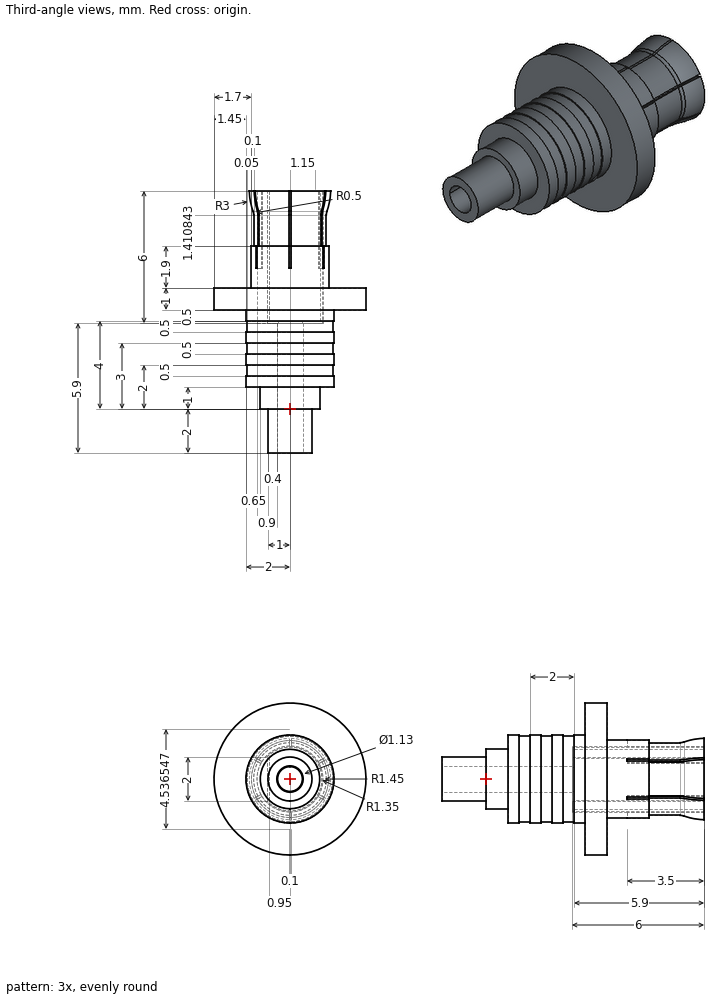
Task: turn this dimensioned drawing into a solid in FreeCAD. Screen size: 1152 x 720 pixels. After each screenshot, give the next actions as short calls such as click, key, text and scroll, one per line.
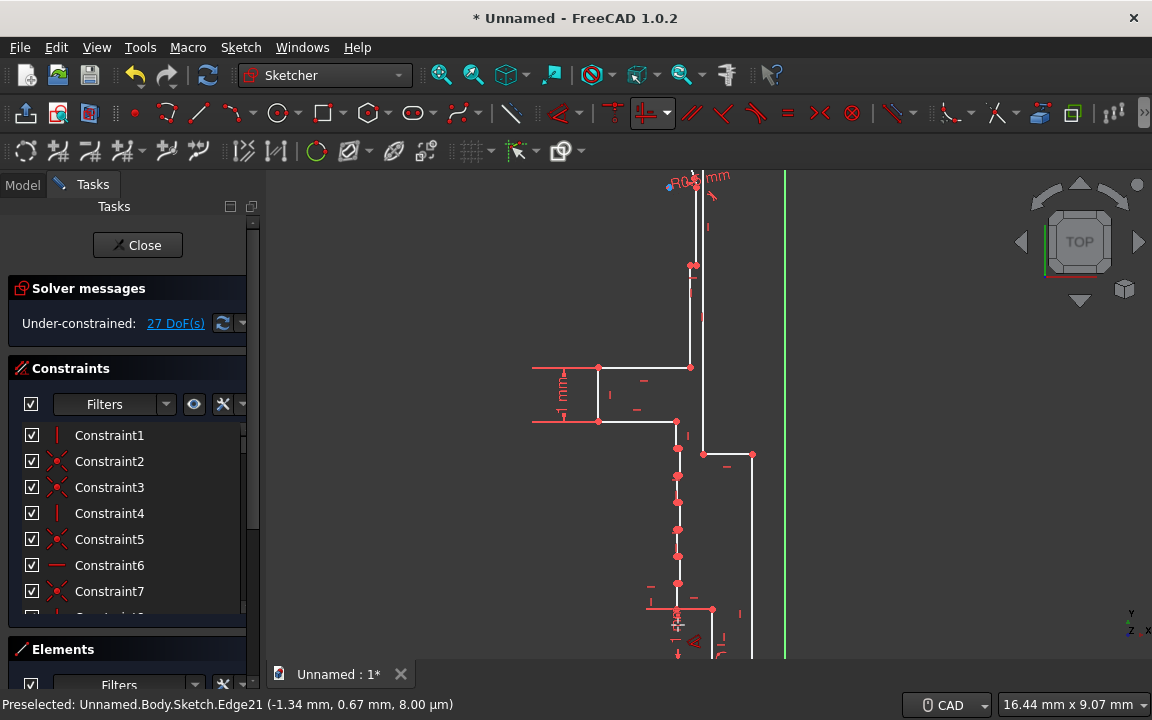
scroll(599, 385, down, 4)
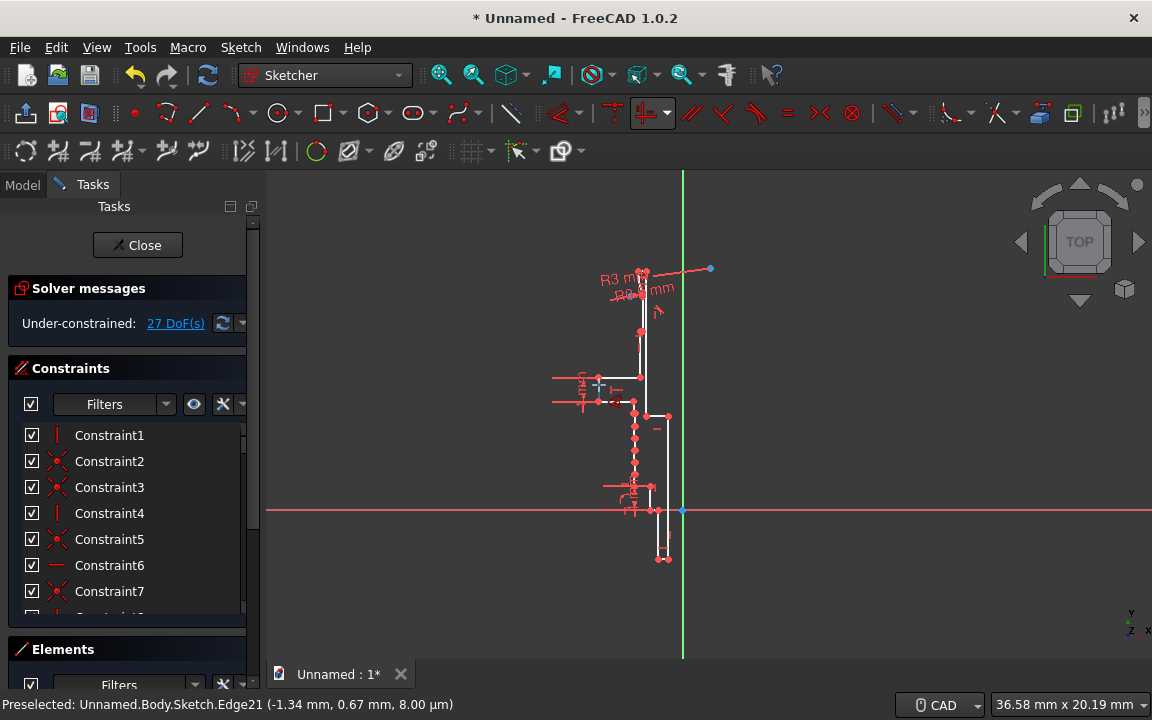
scroll(658, 525, up, 2)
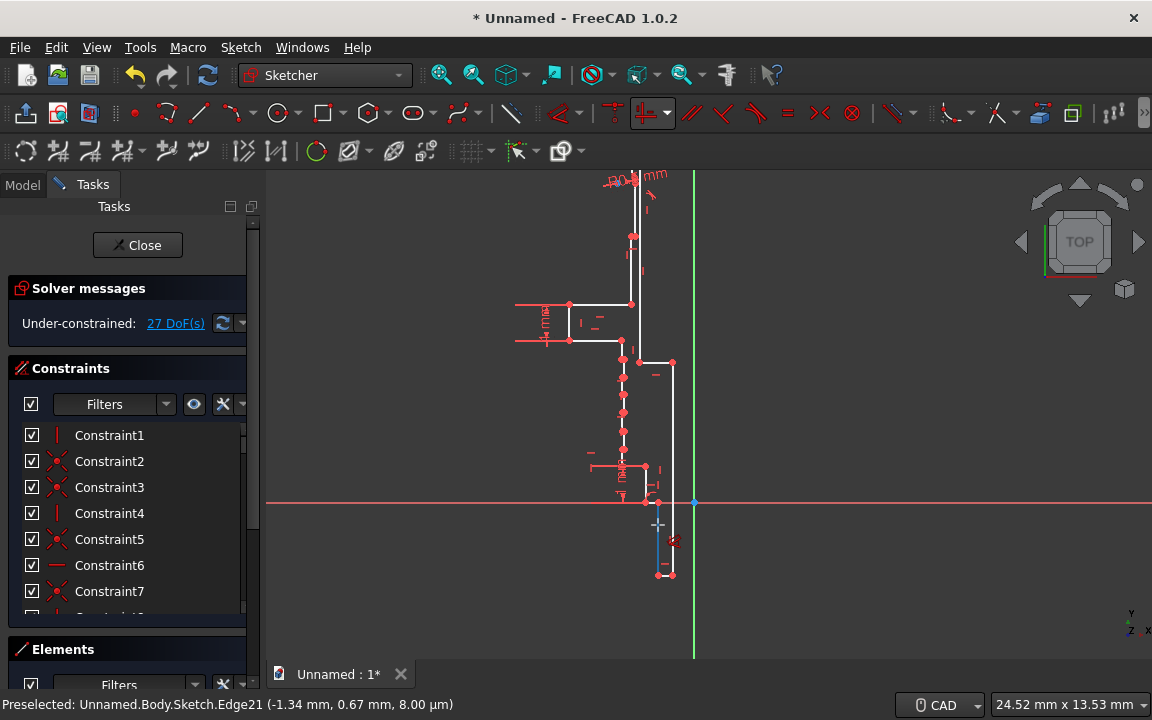
click(658, 525)
click(624, 539)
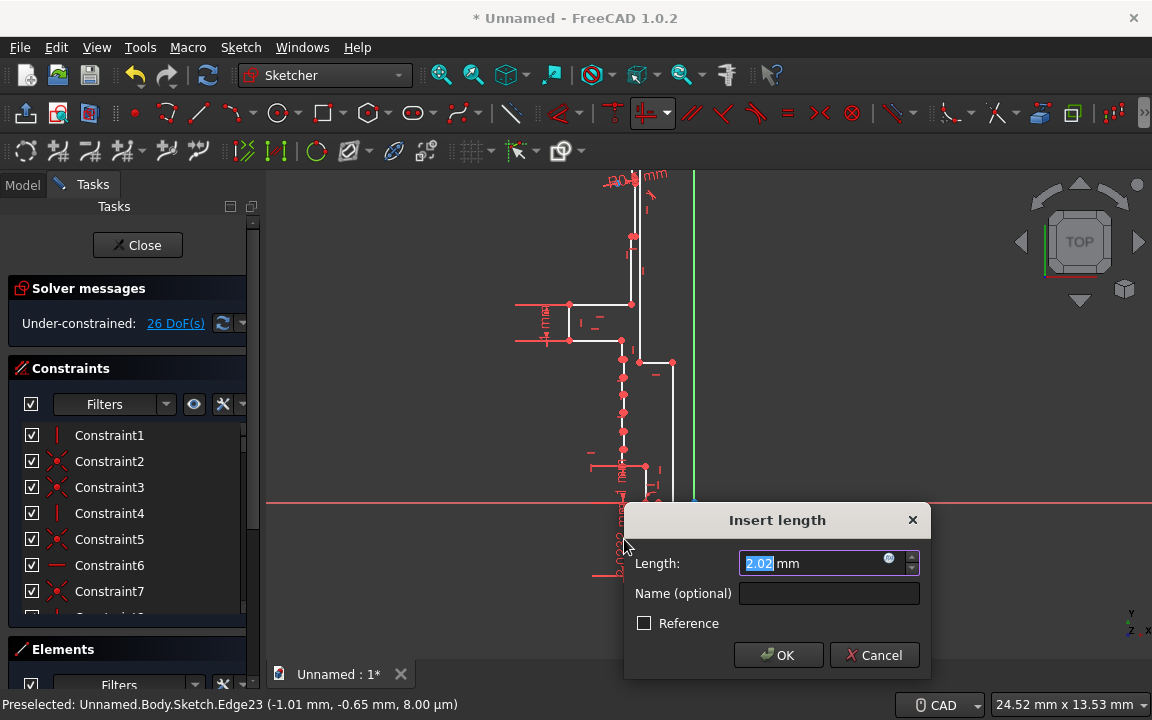
text(2)
key(Return)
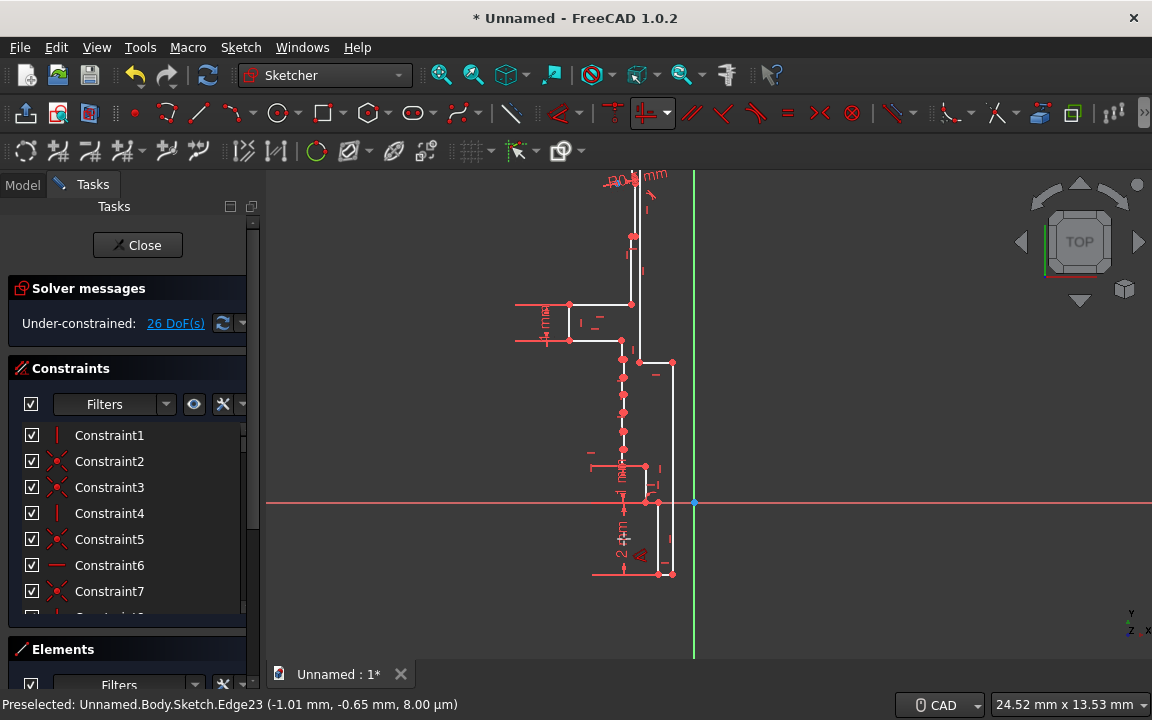
click(640, 319)
click(674, 280)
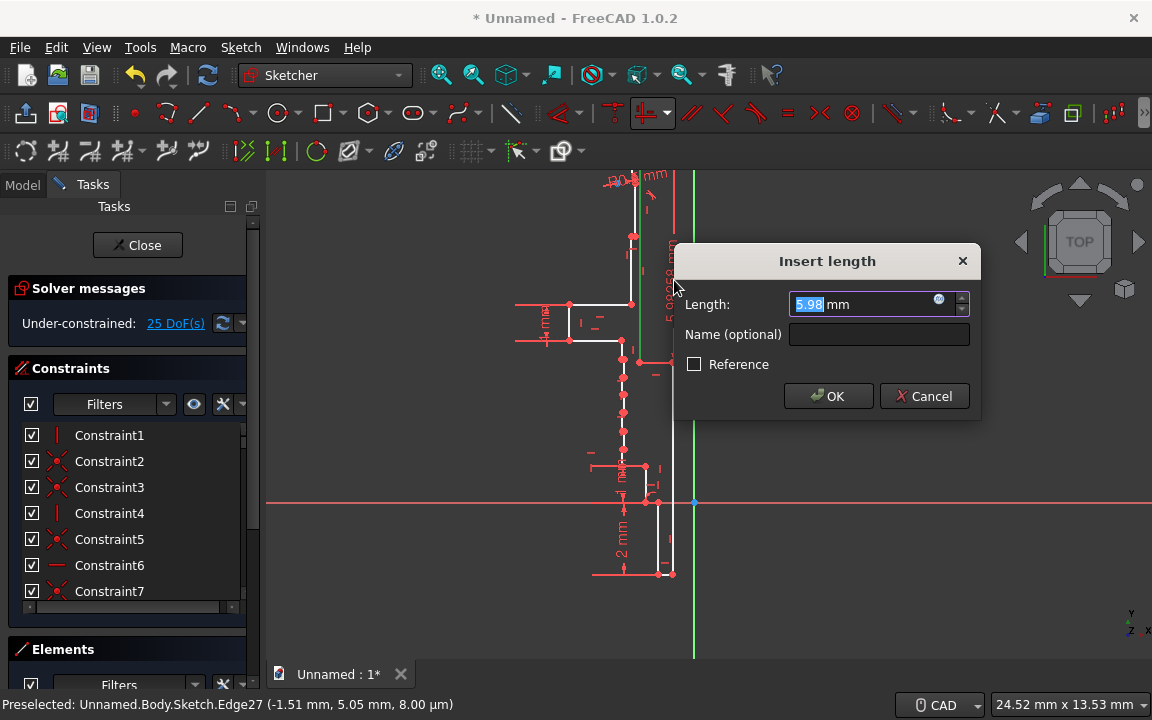
text(6)
key(Return)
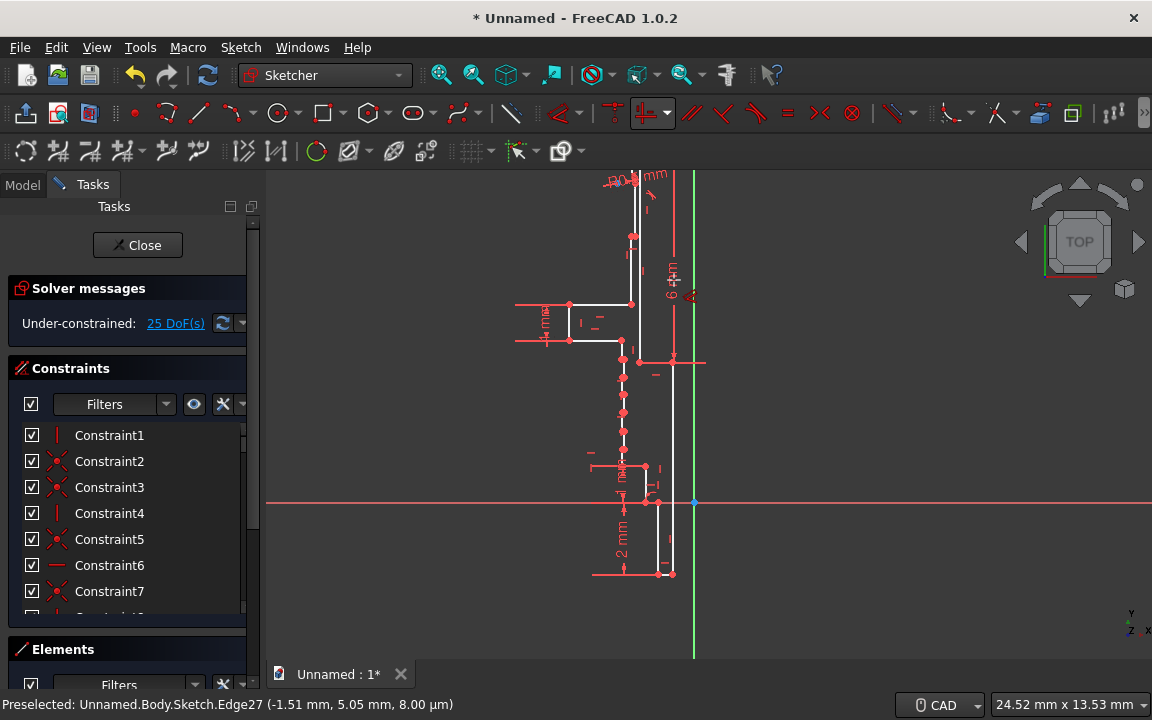
click(622, 341)
click(658, 307)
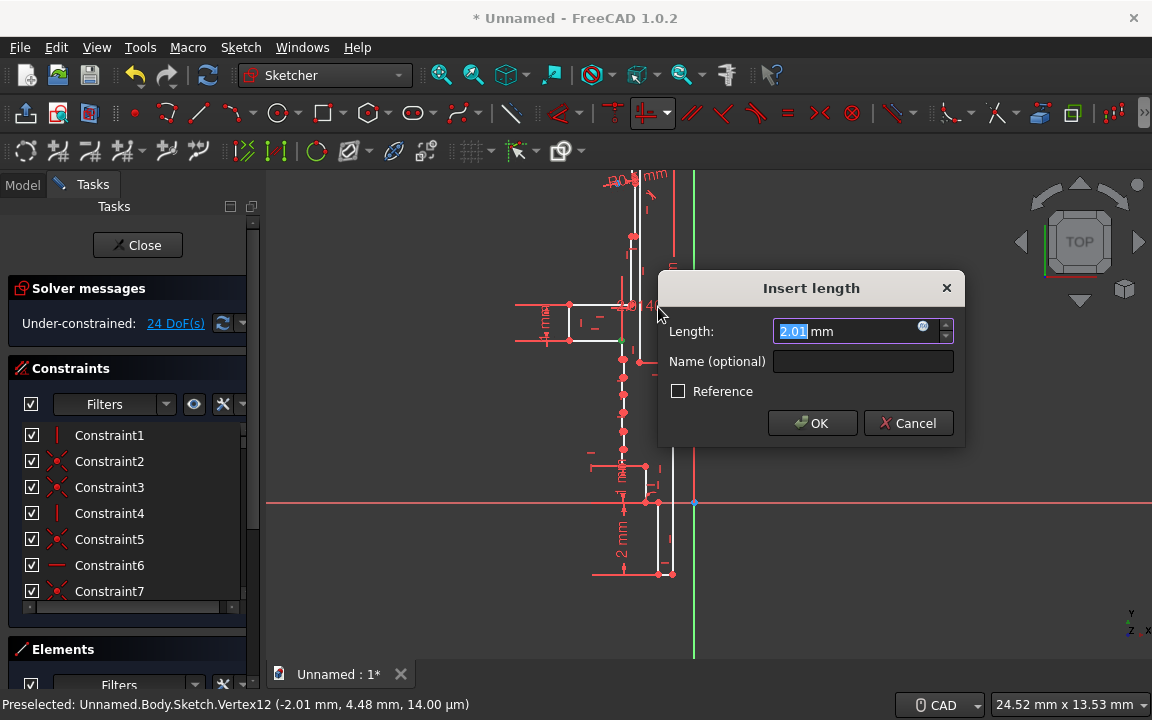
text(2)
key(Return)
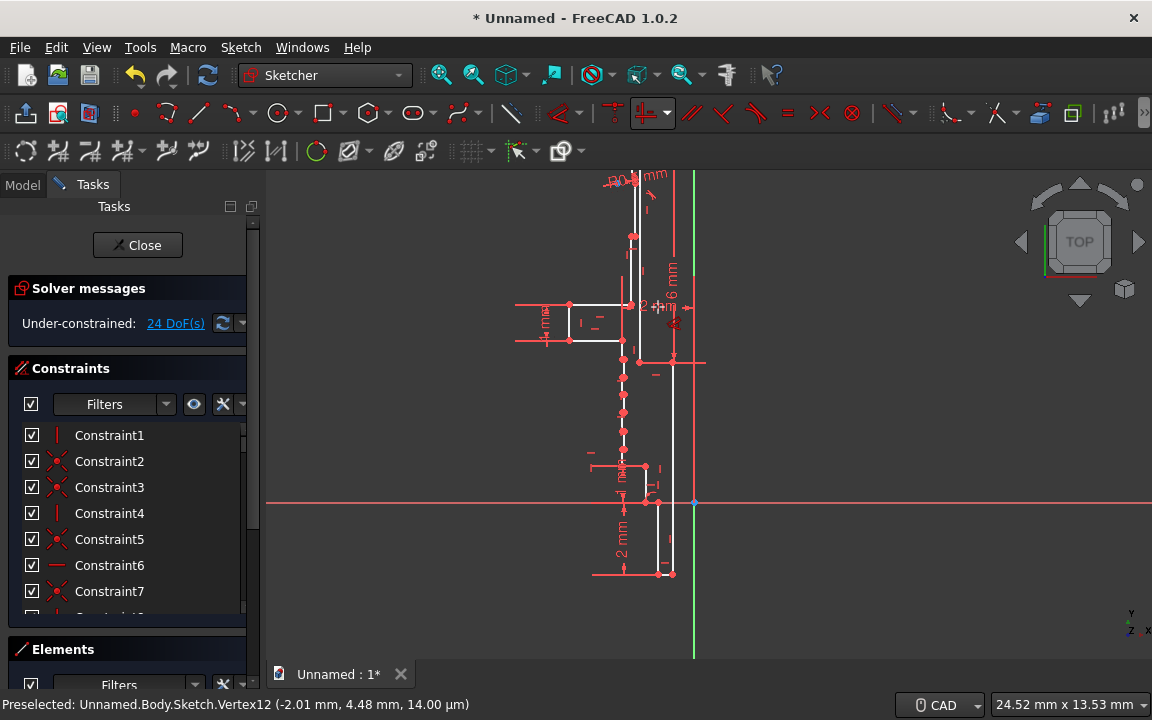
scroll(622, 359, up, 10)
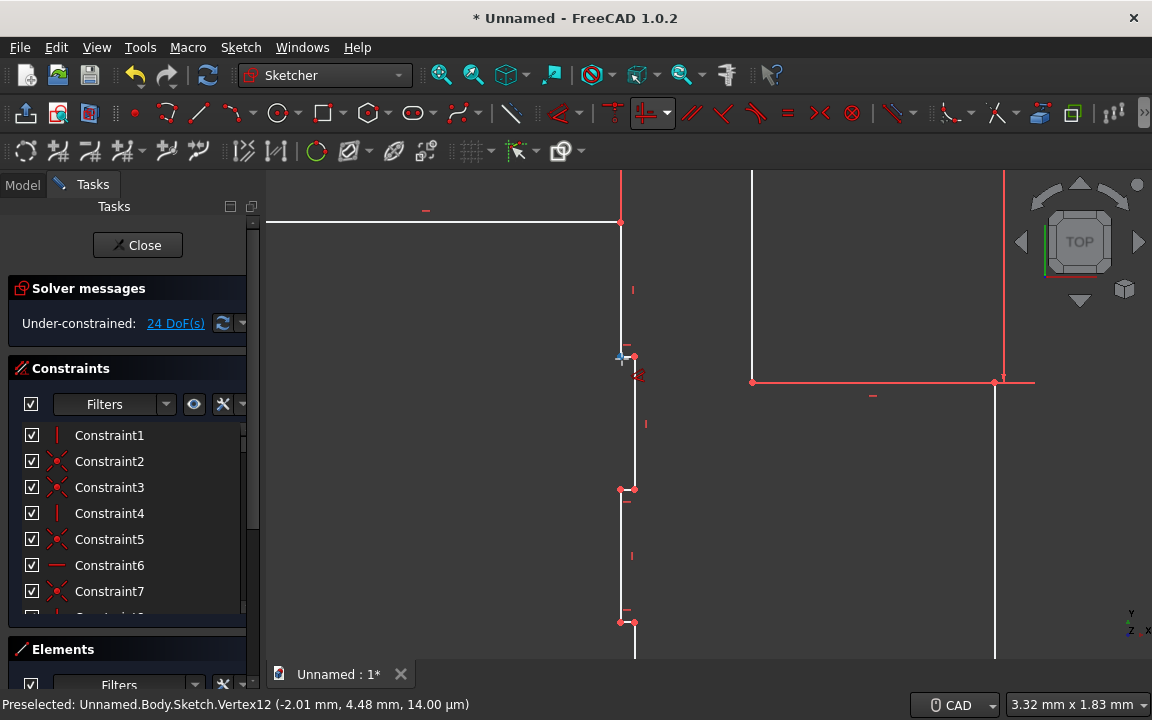
click(621, 357)
click(587, 494)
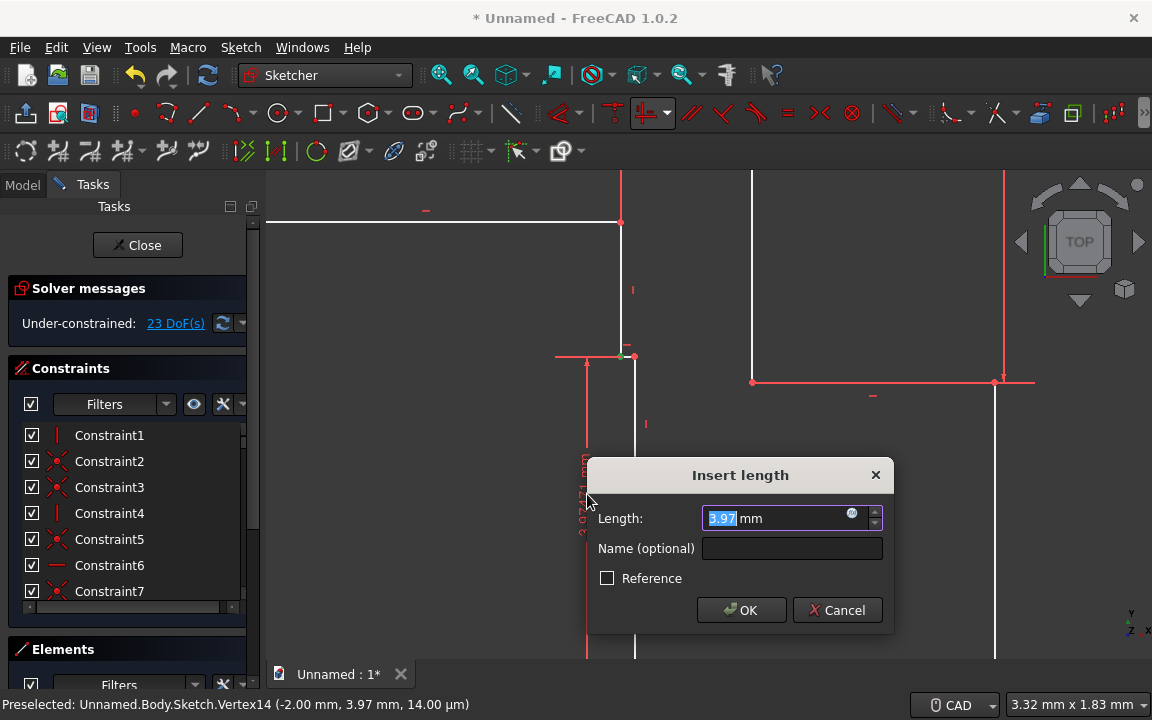
text(4)
key(Return)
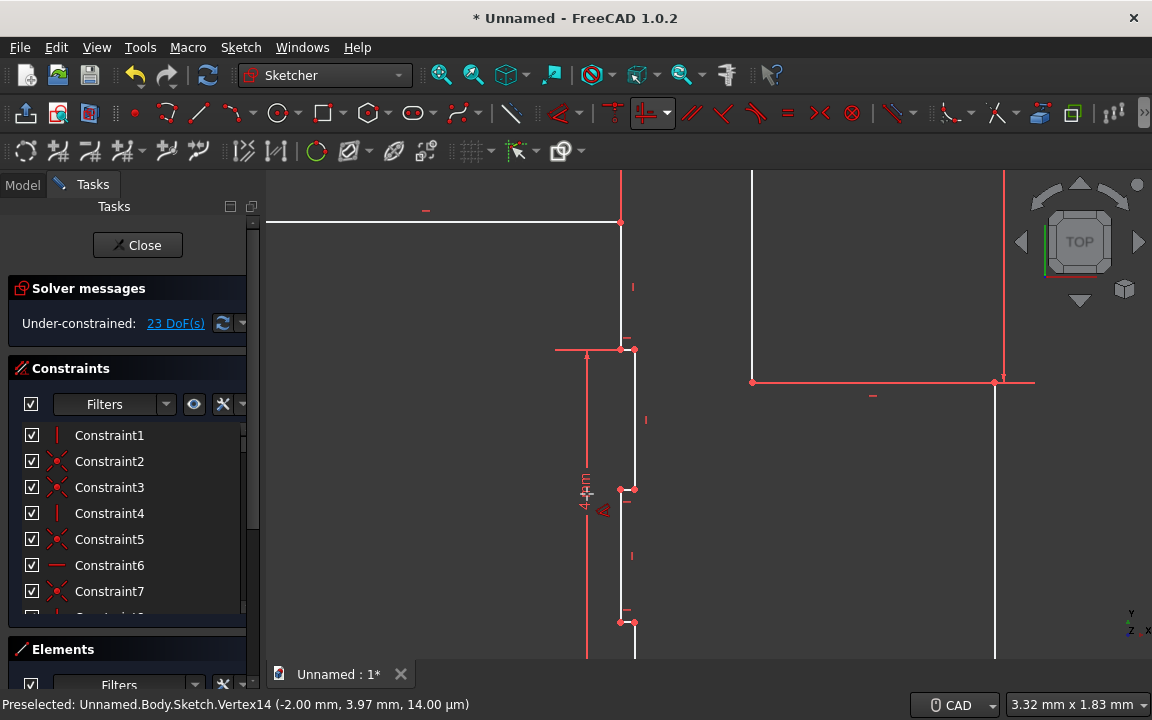
click(621, 490)
click(804, 456)